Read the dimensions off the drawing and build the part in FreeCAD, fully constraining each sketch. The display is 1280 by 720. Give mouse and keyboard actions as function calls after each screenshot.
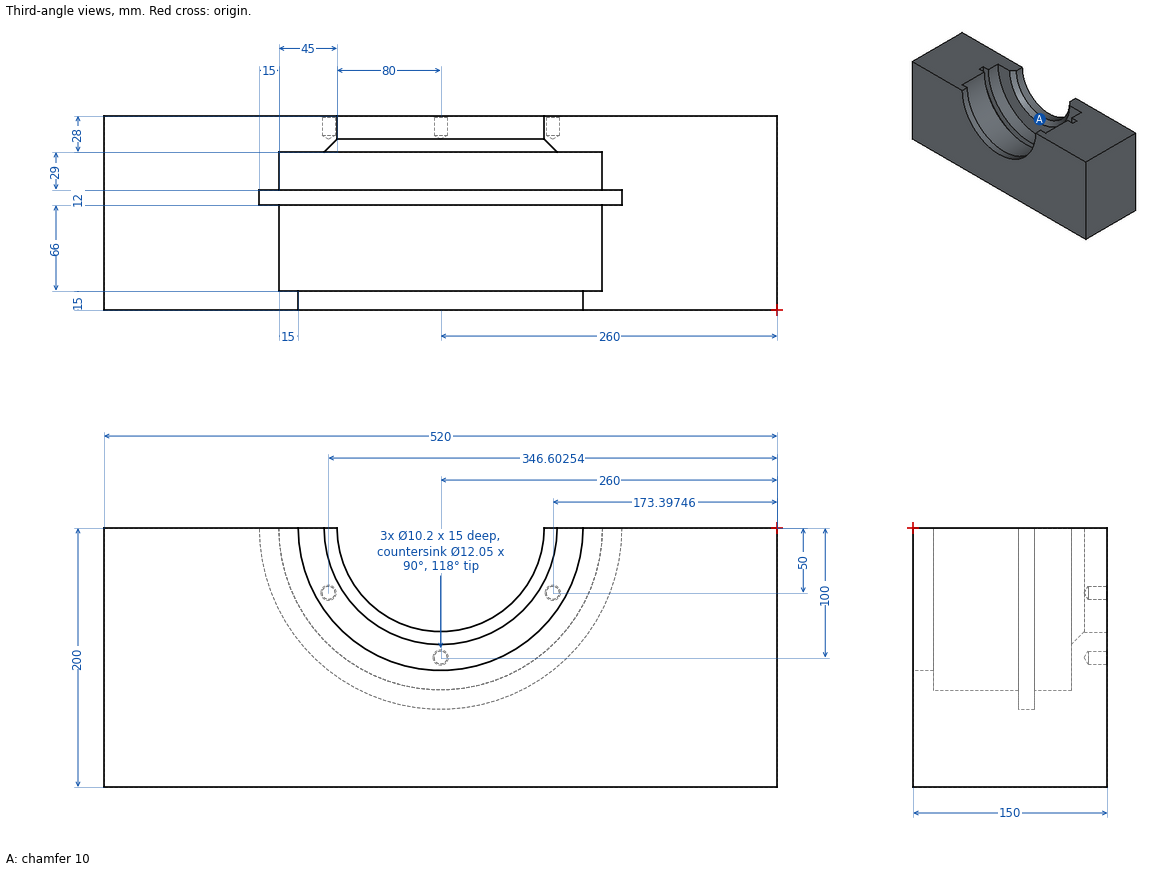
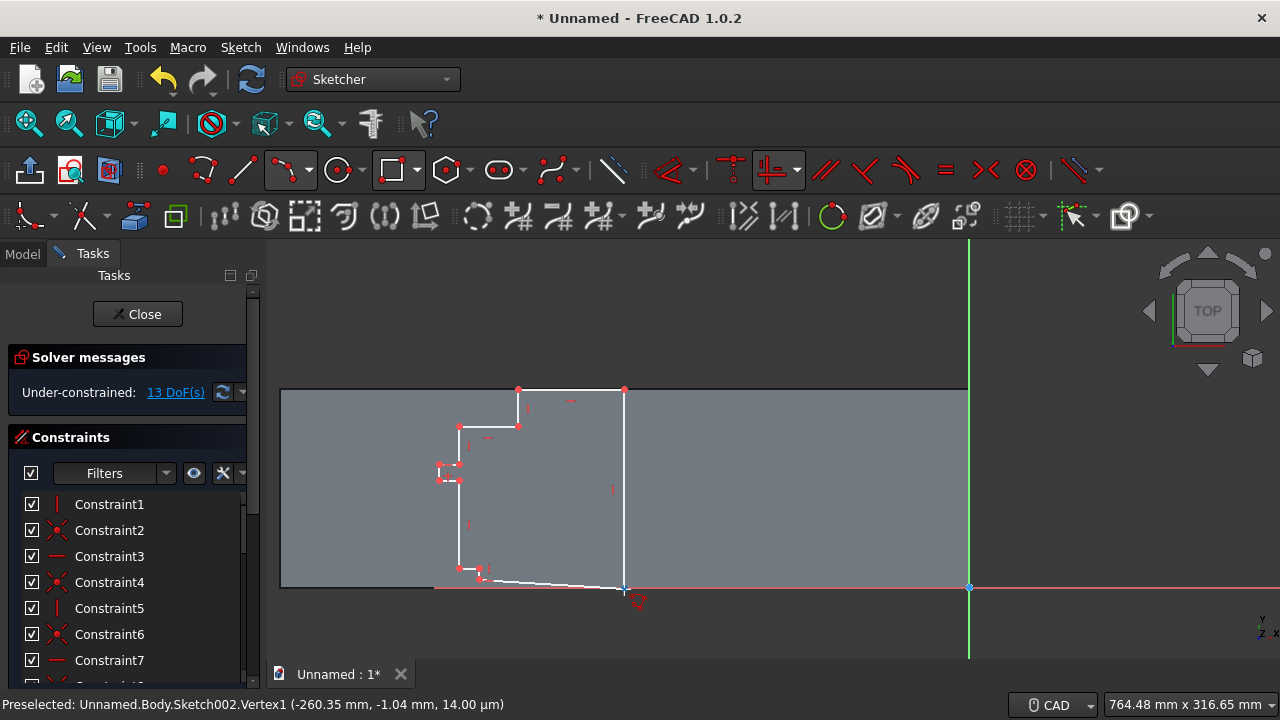
click(244, 170)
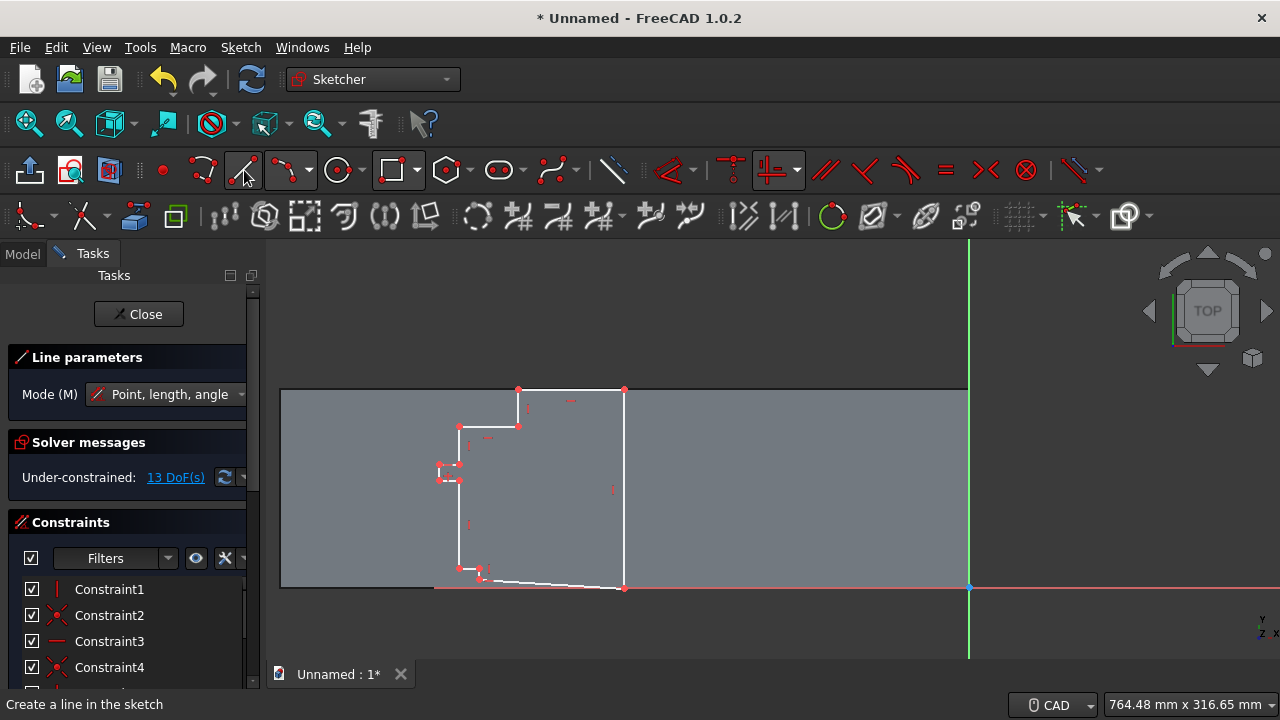
click(624, 369)
click(624, 309)
key(Escape)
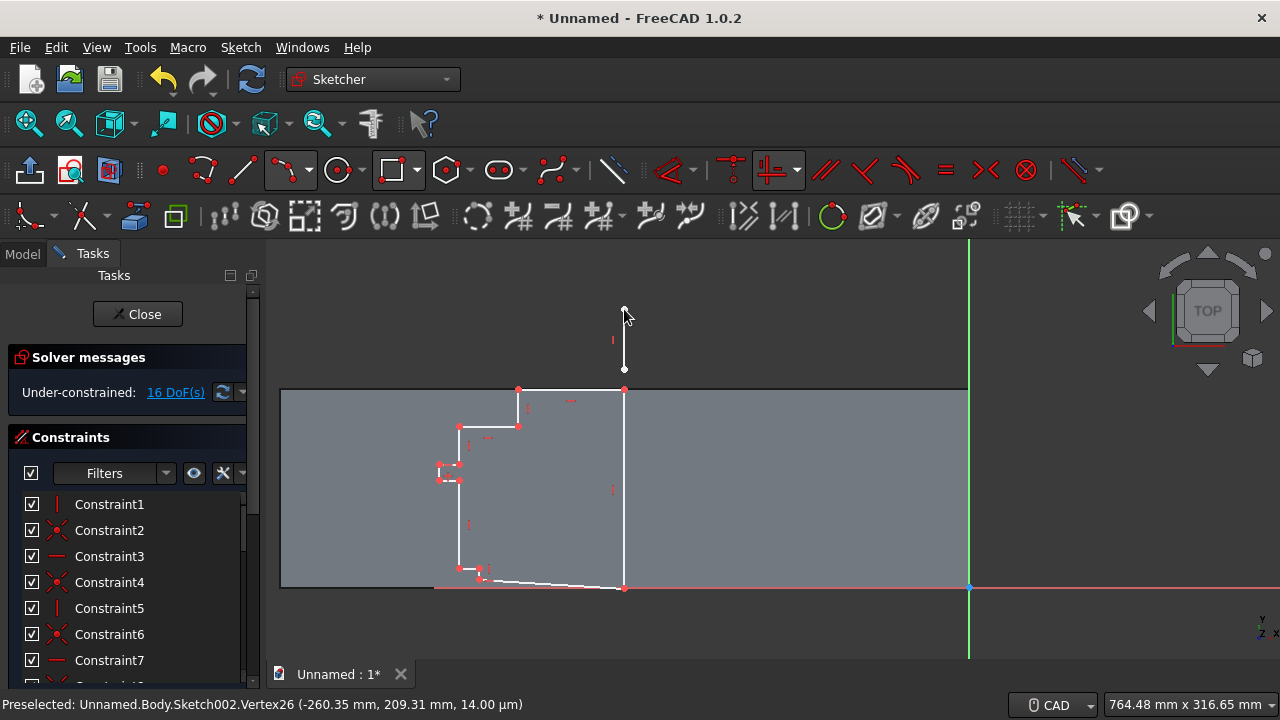
click(624, 352)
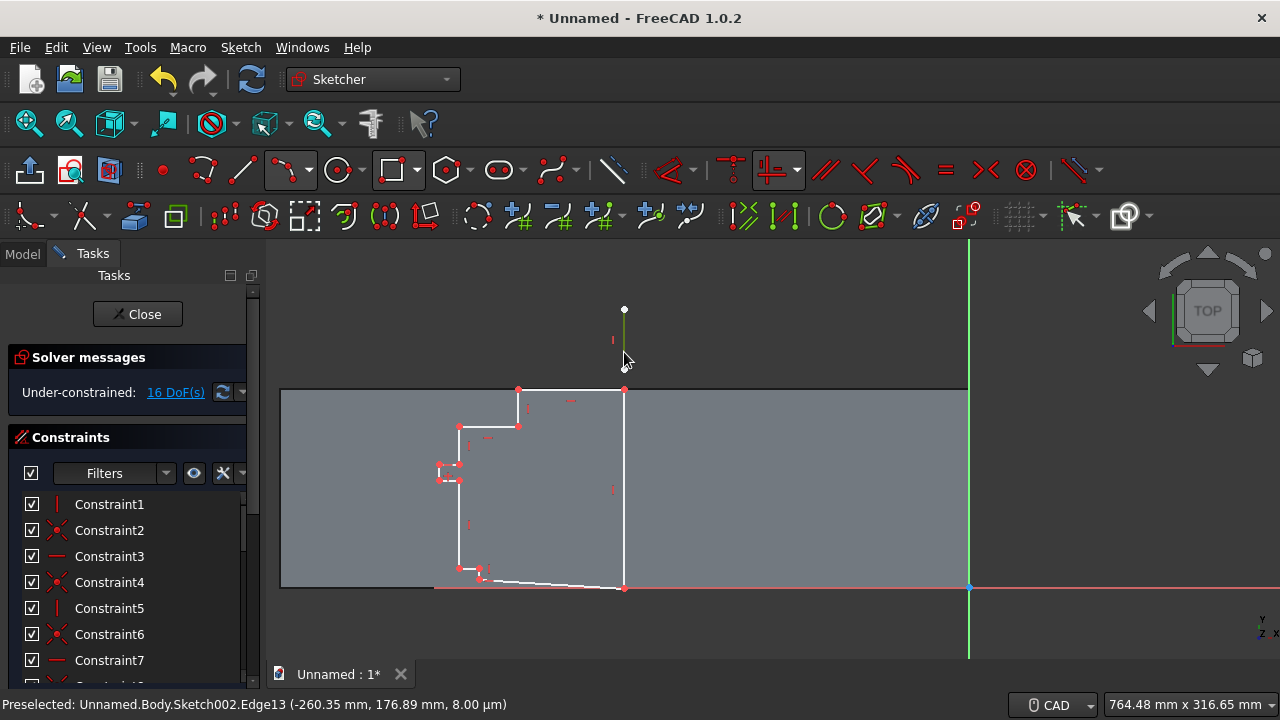
key(g)
key(n)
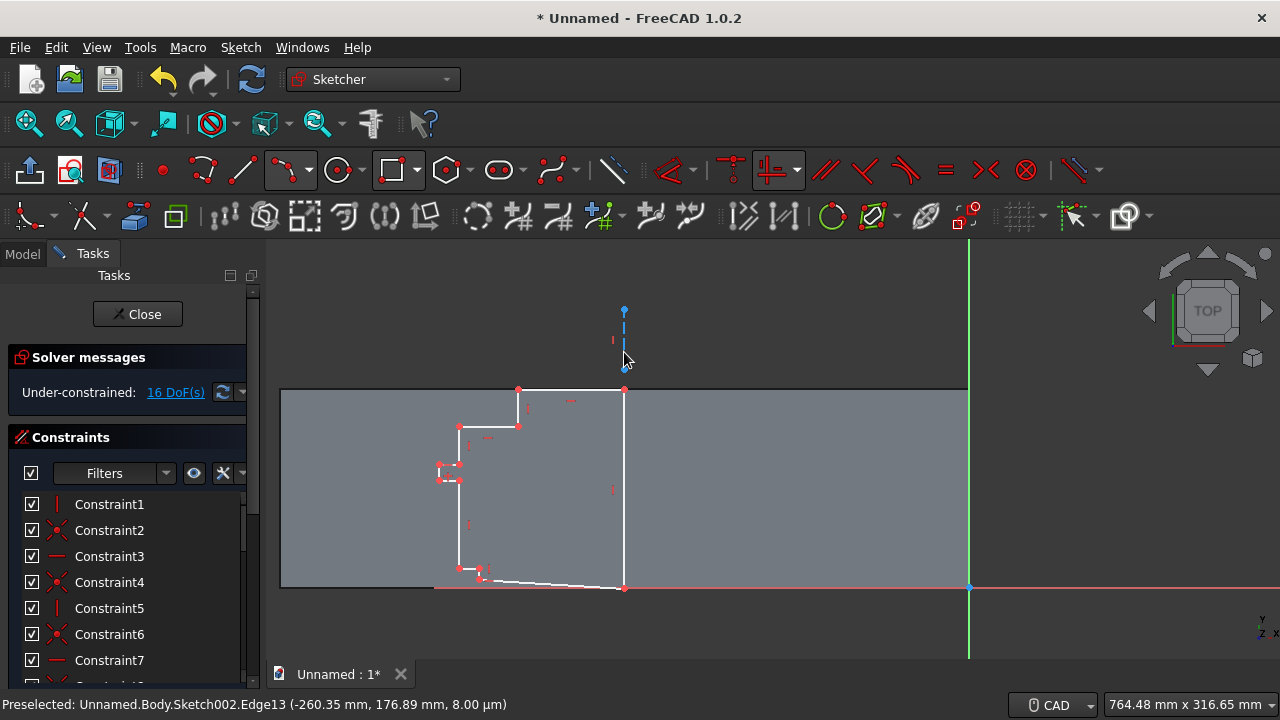
click(581, 586)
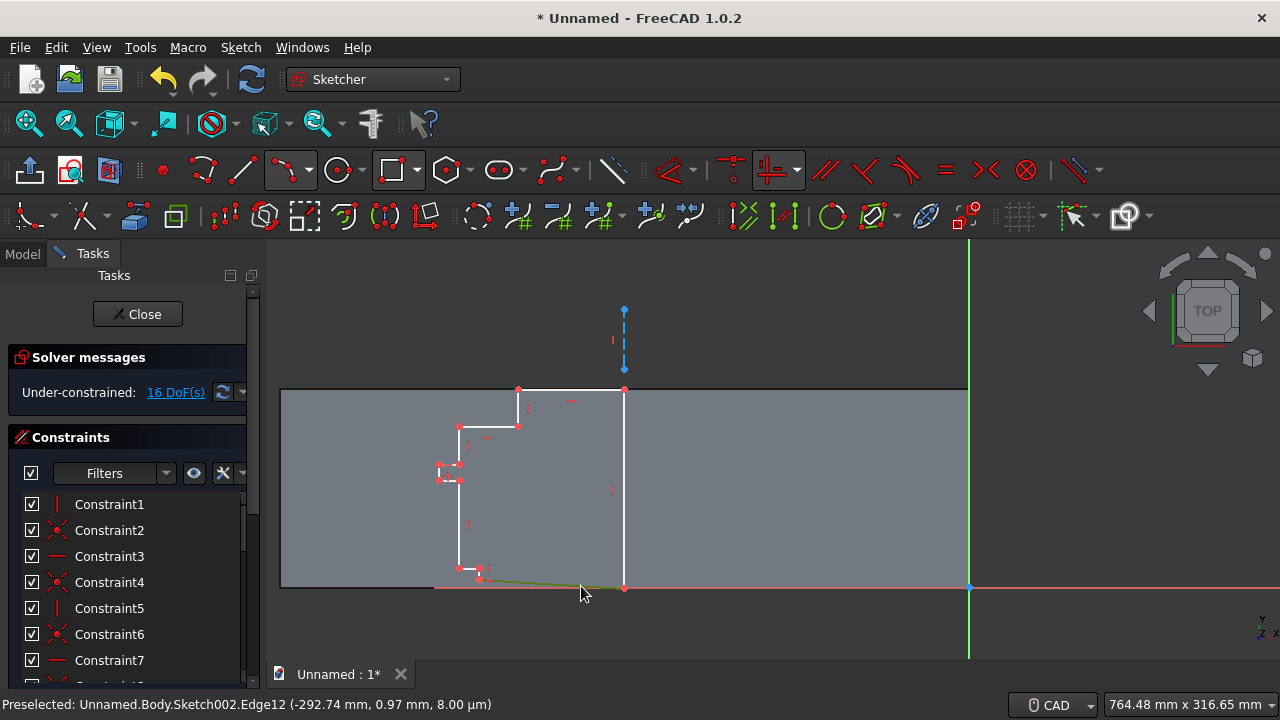
click(800, 170)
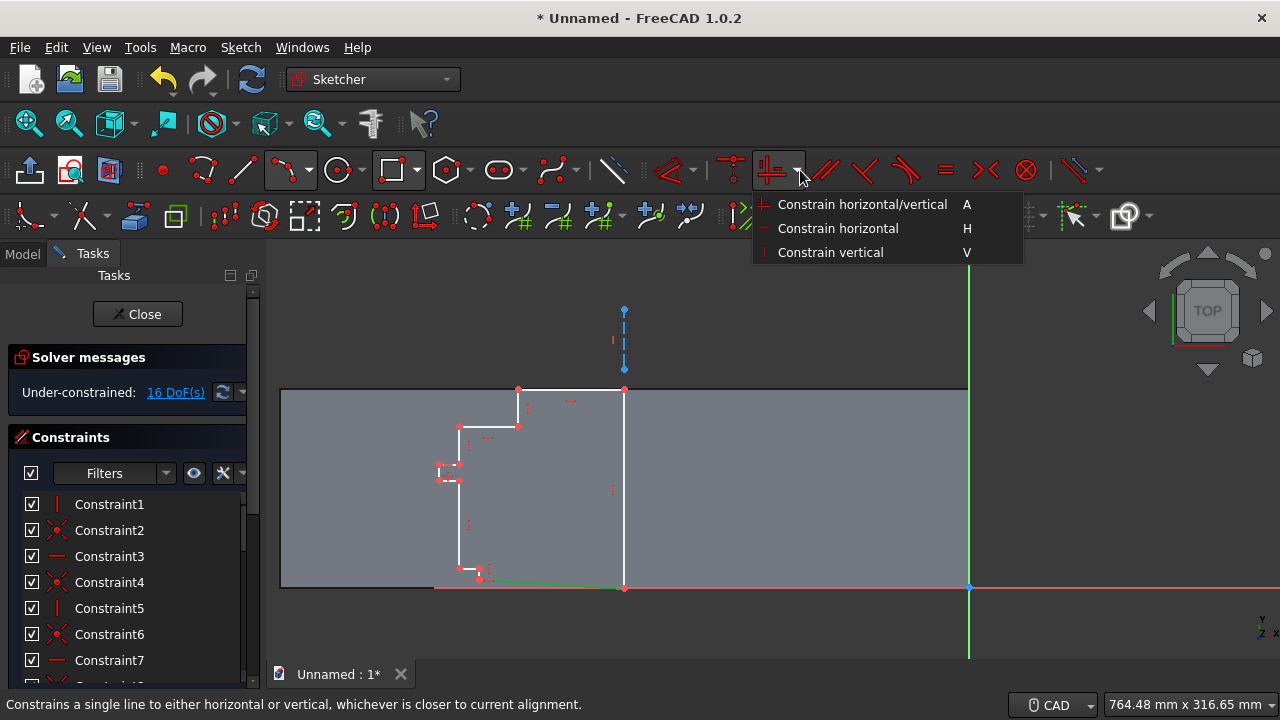
click(888, 228)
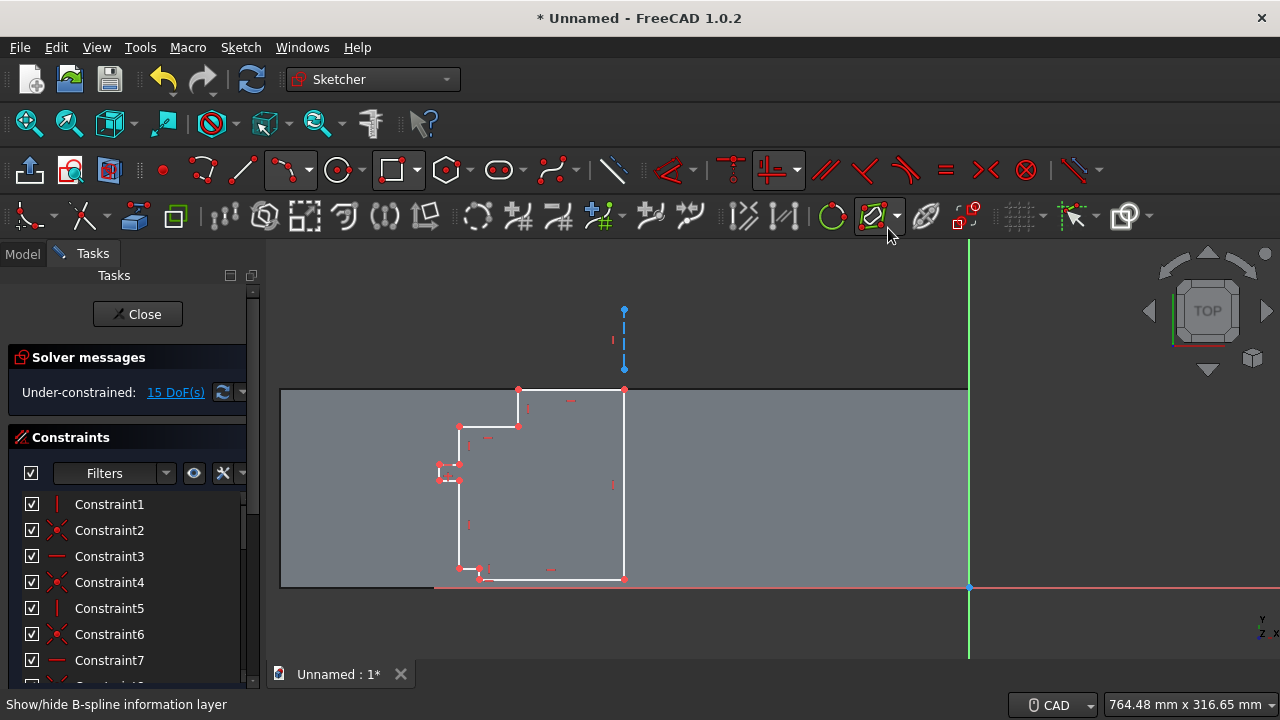
click(624, 580)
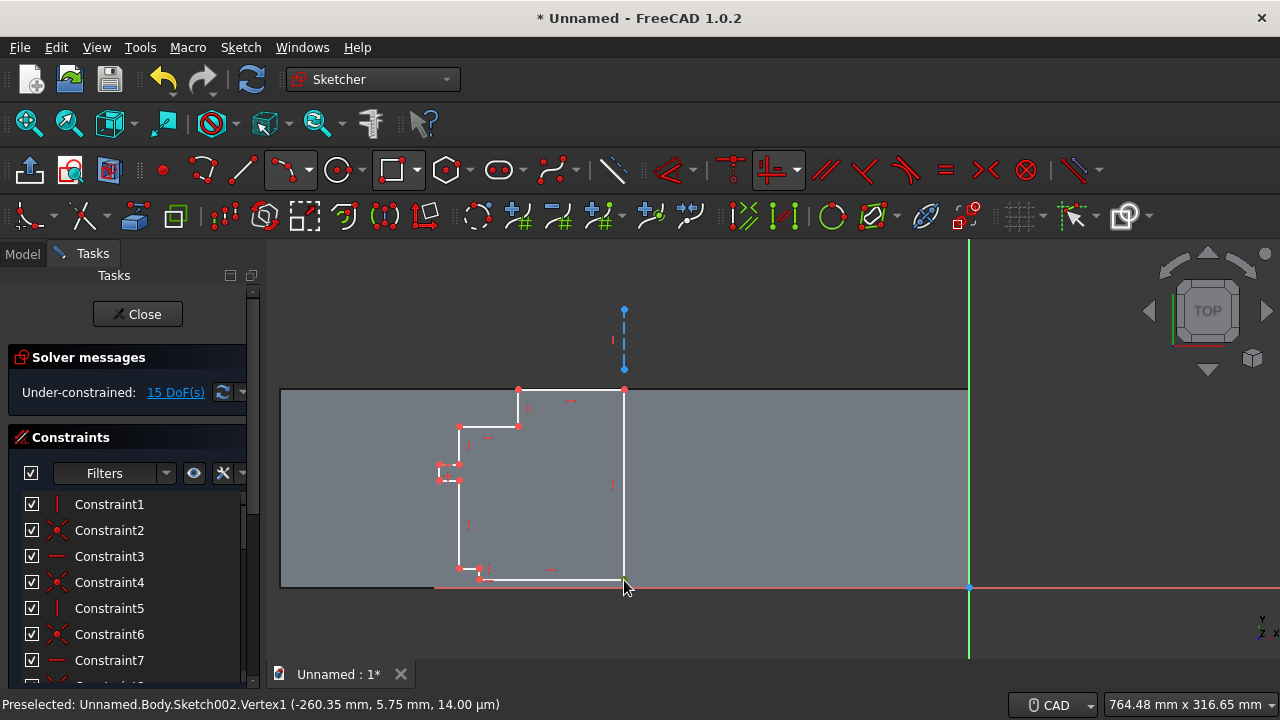
click(704, 588)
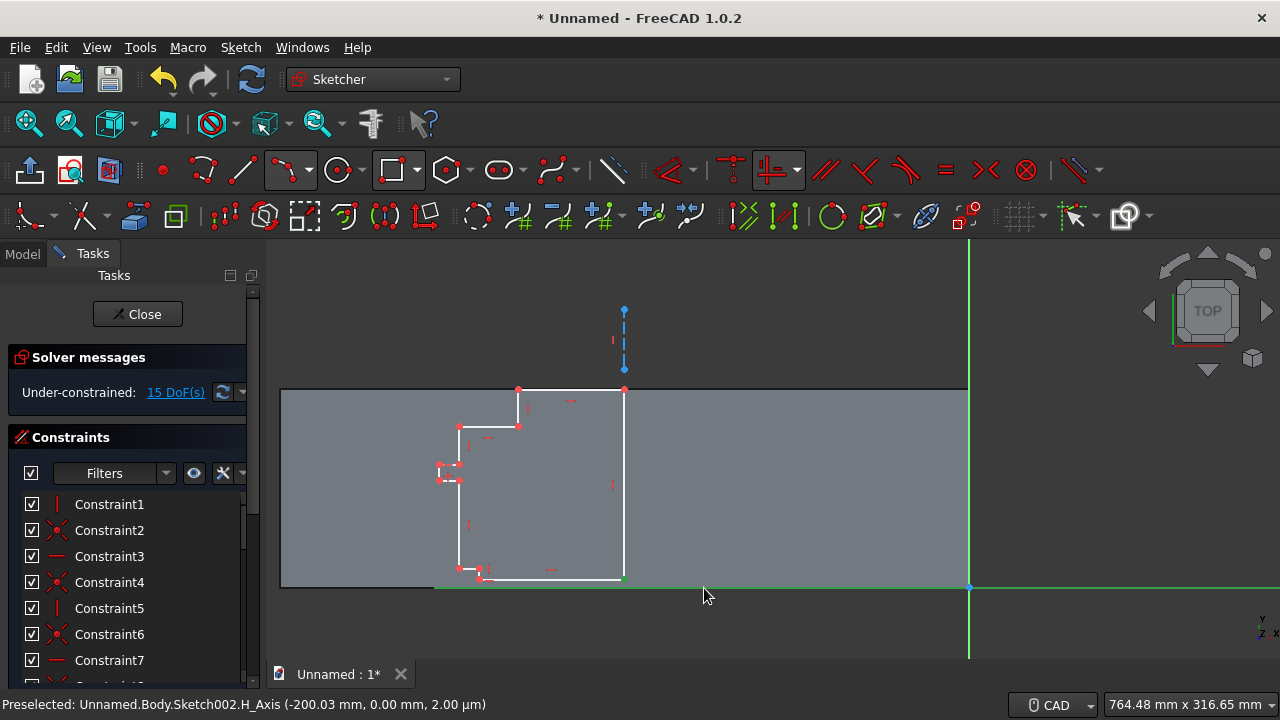
click(732, 170)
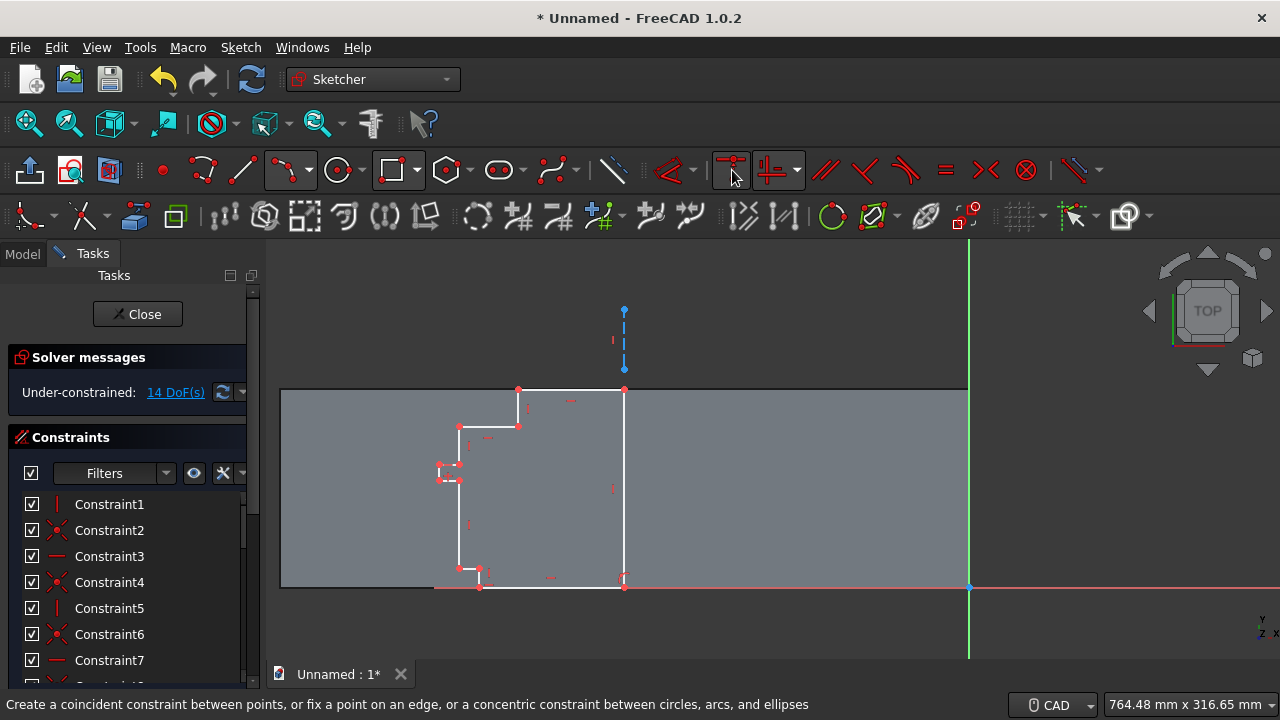
click(668, 170)